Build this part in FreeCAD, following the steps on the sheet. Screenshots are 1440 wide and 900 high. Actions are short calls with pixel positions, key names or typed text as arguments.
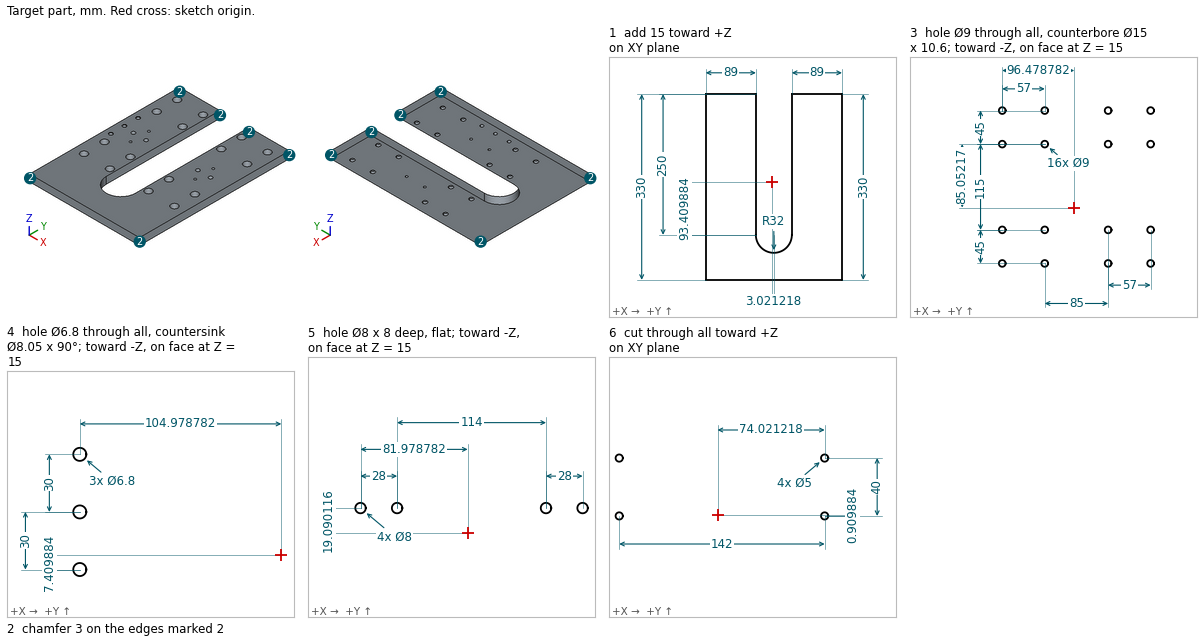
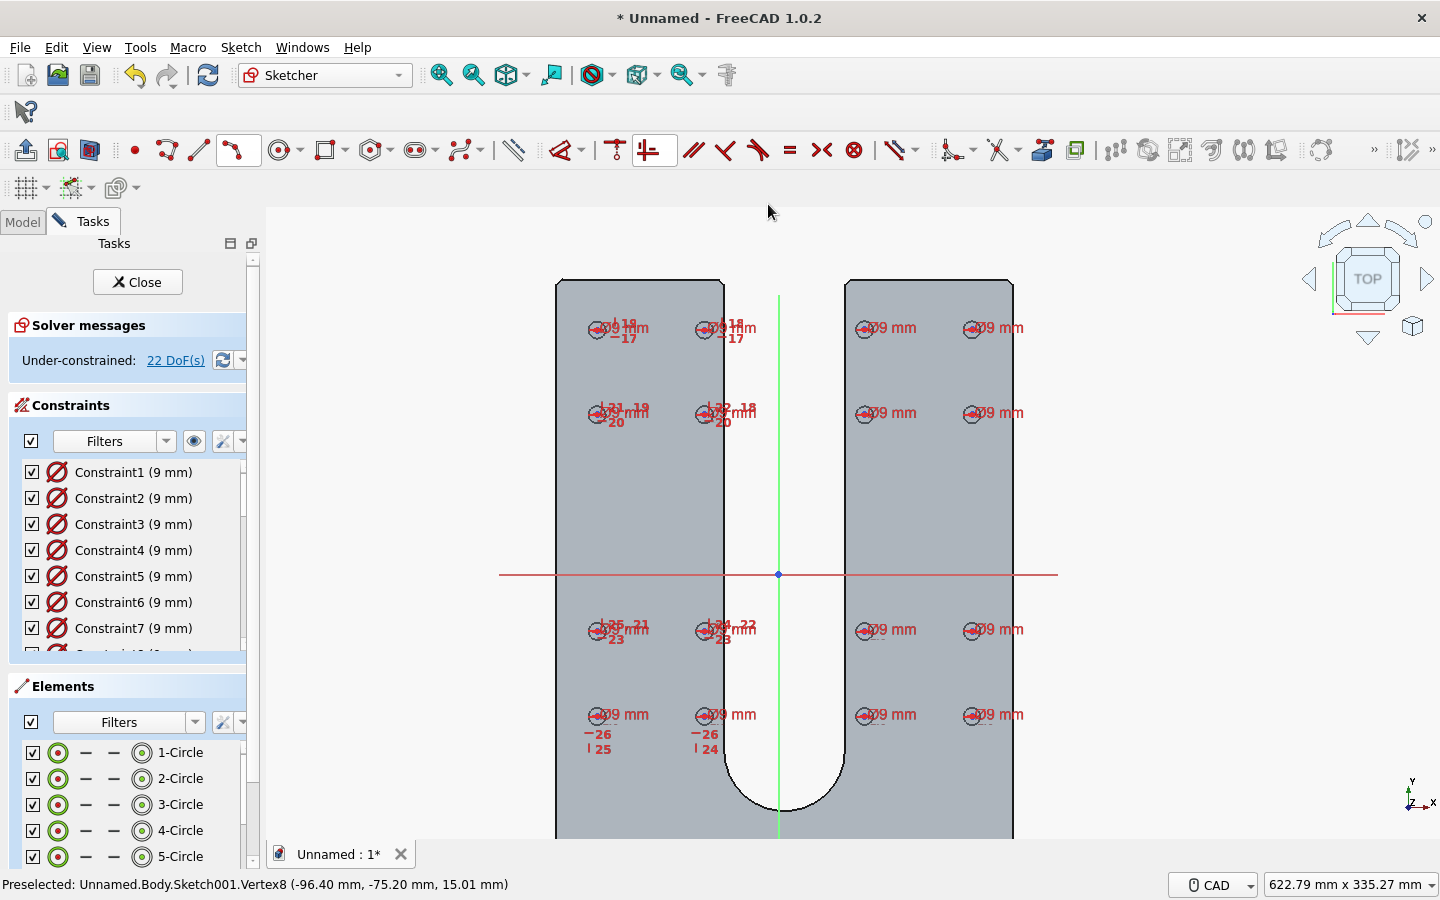
click(705, 717)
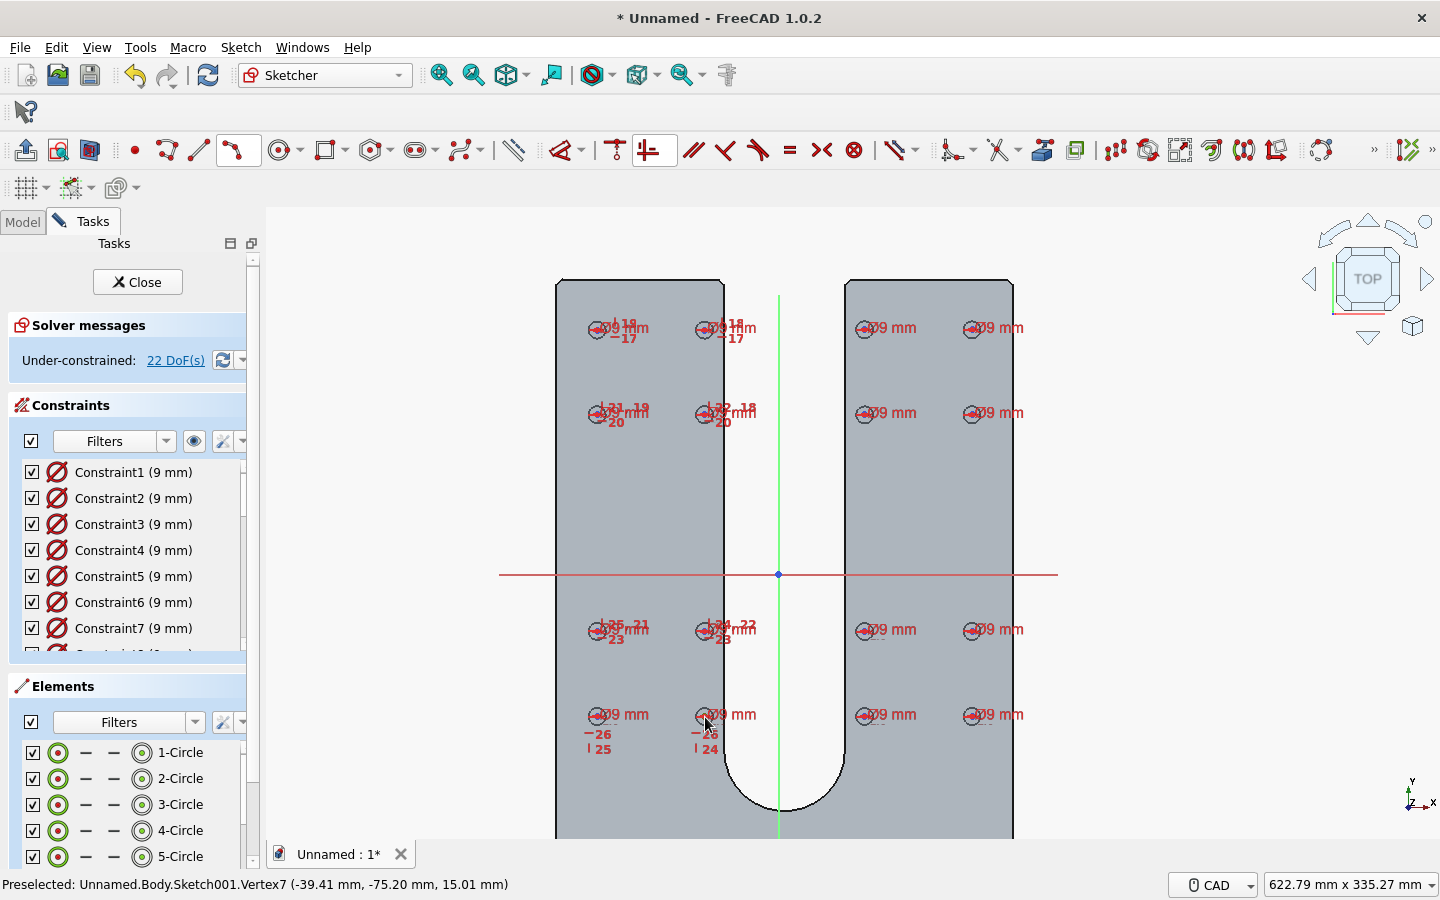
click(865, 717)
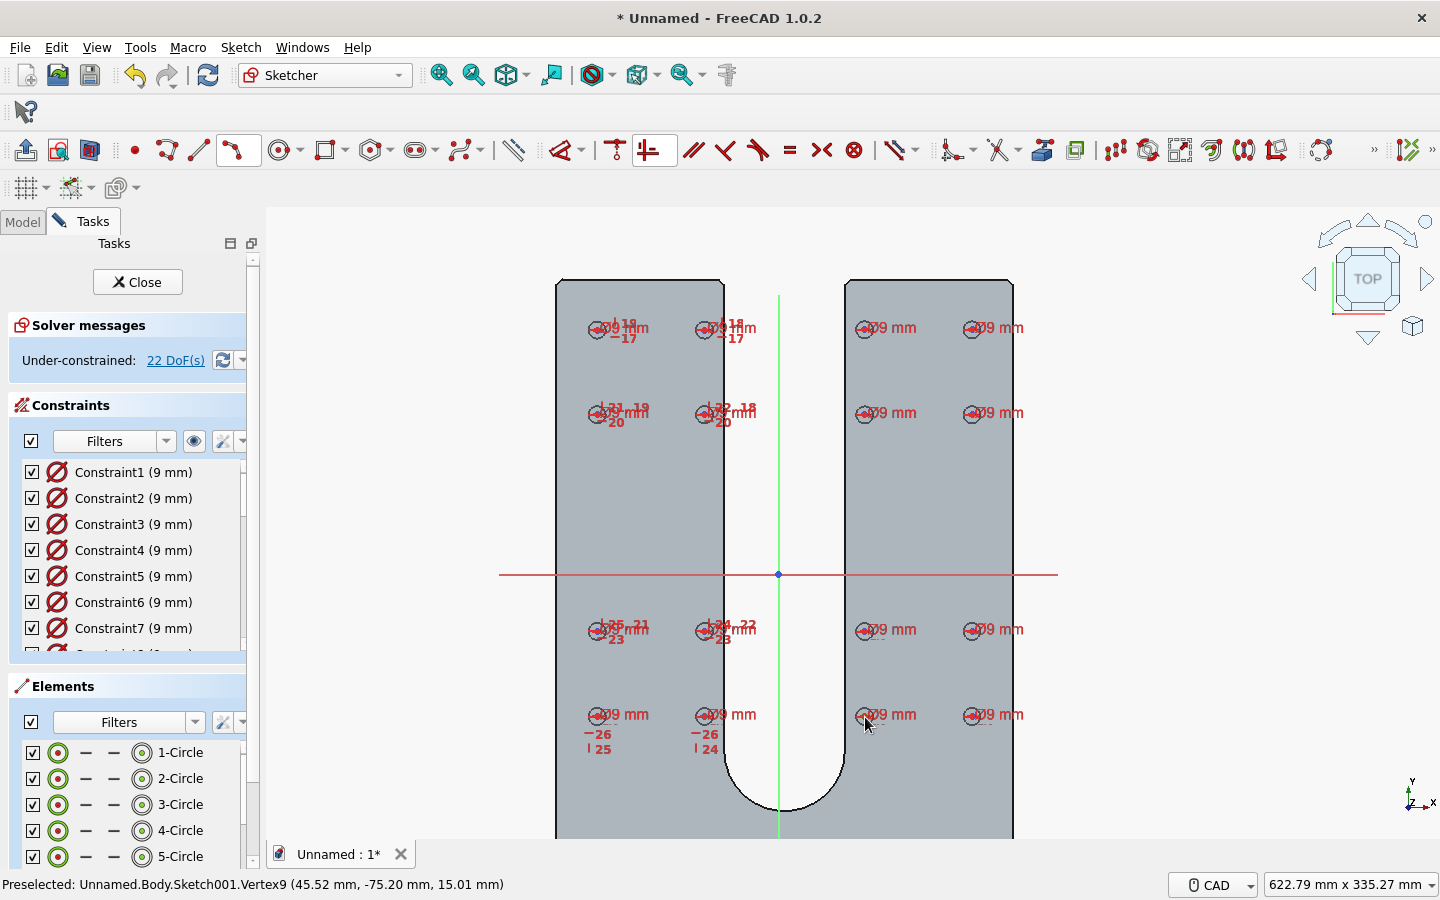
click(672, 150)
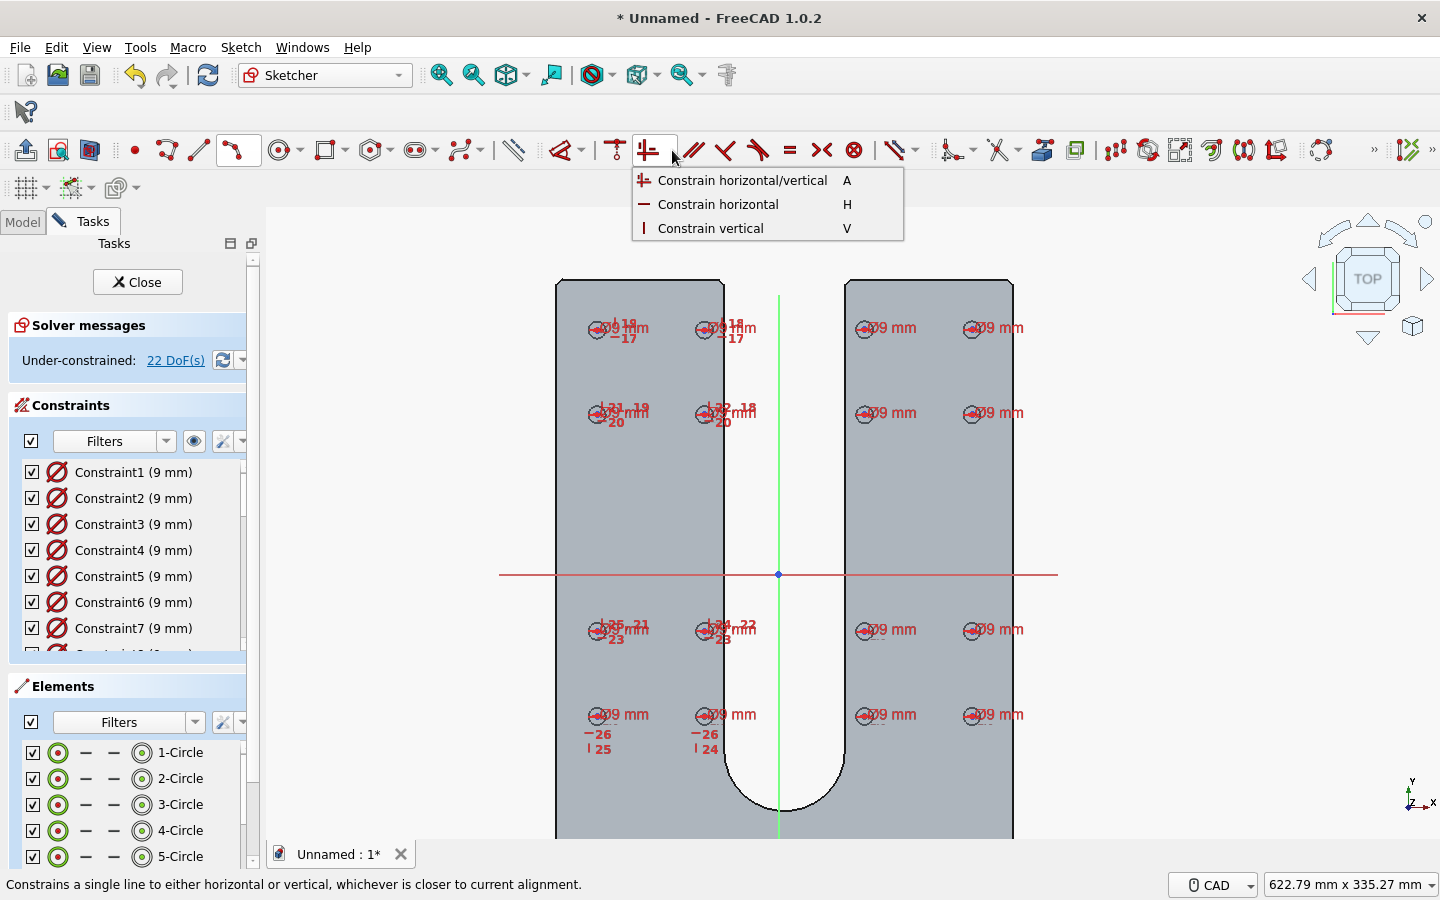
click(768, 204)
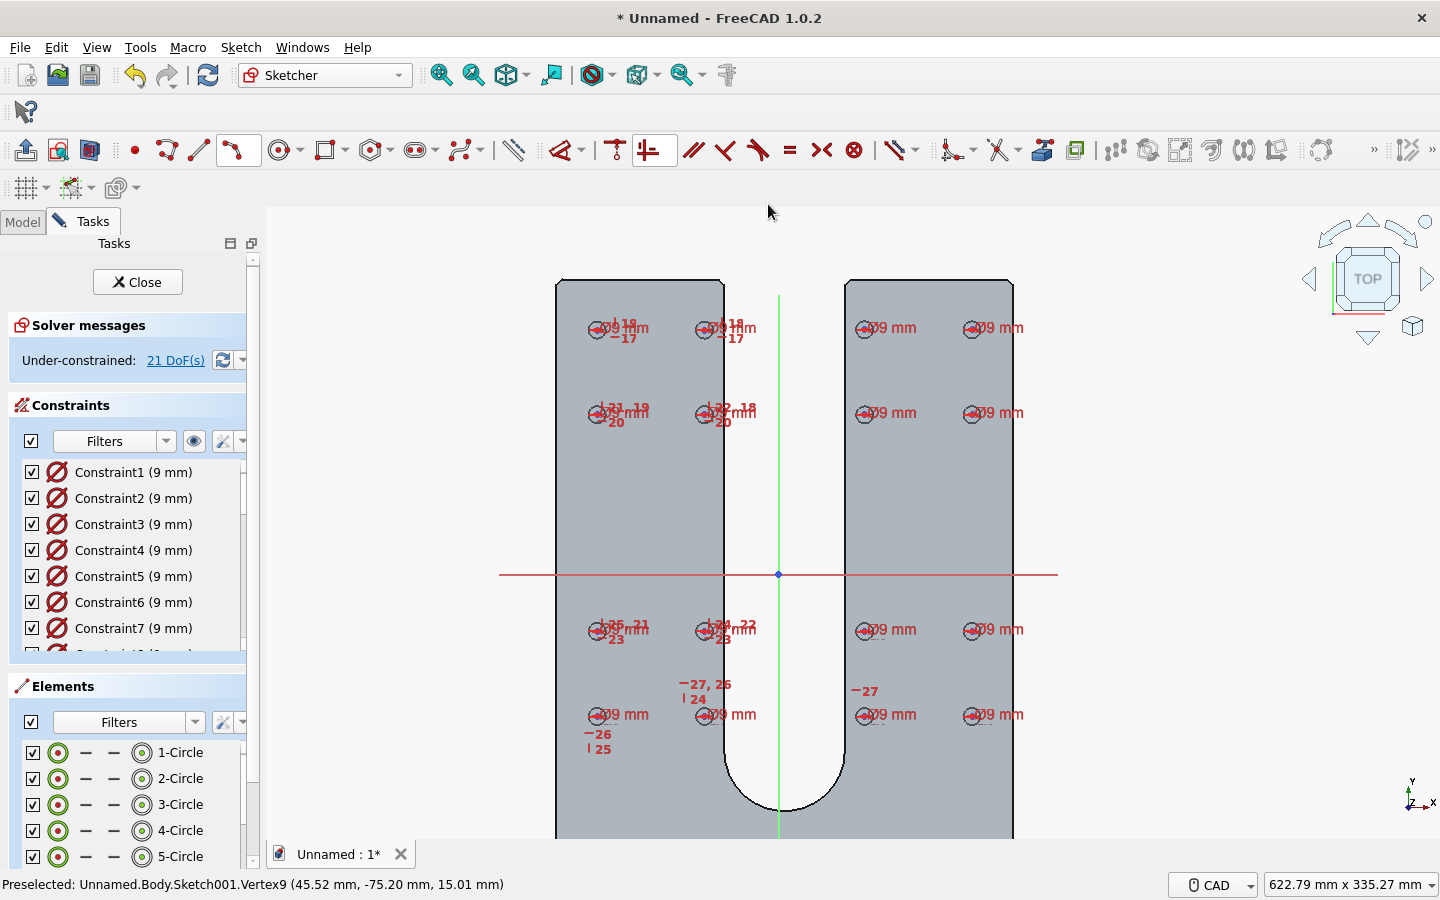
click(865, 717)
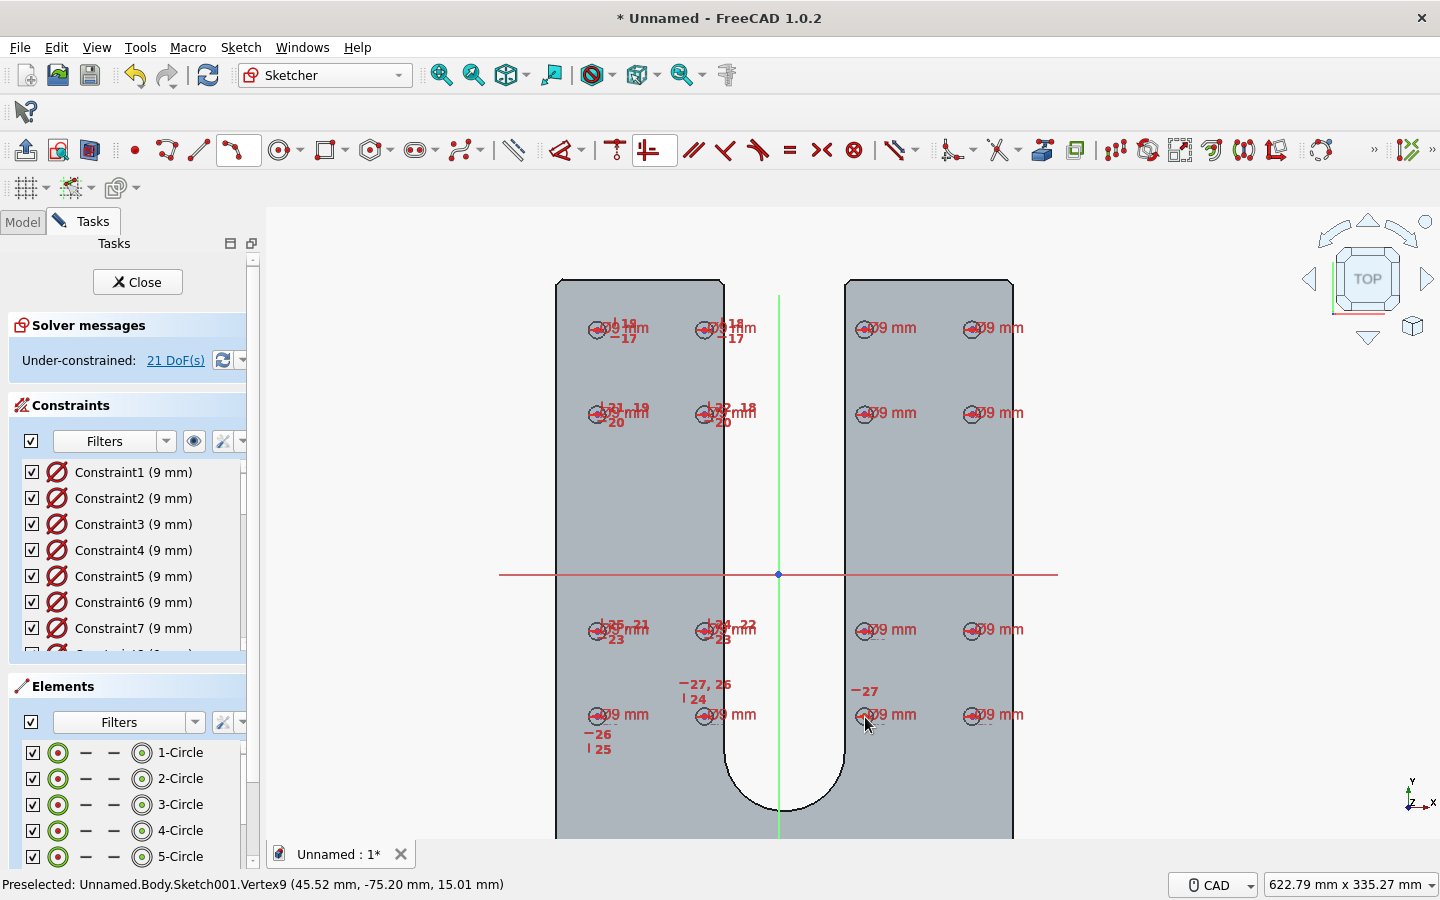
click(865, 632)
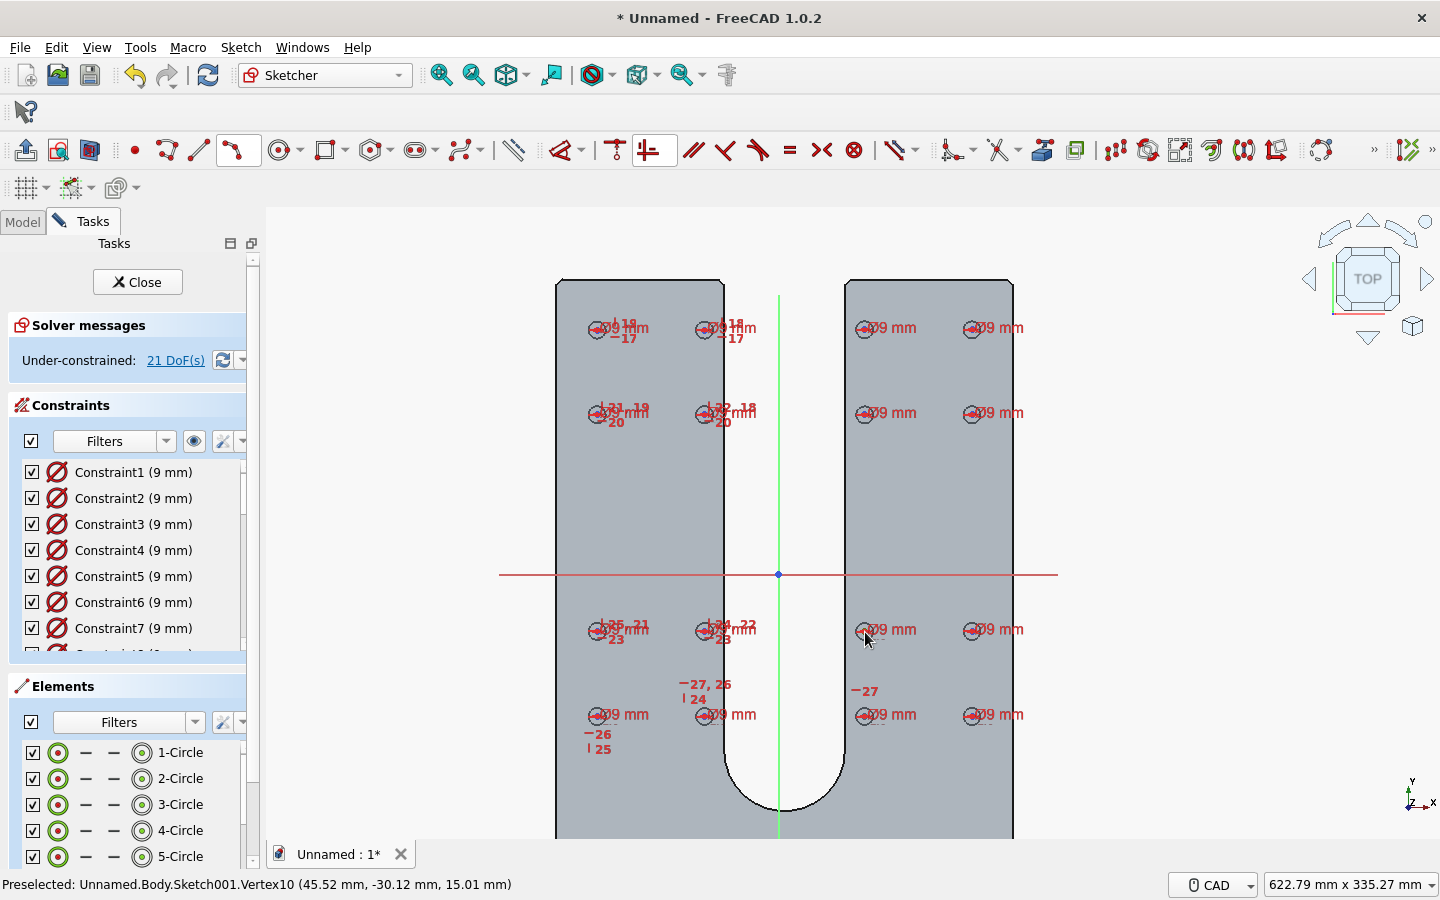
click(672, 150)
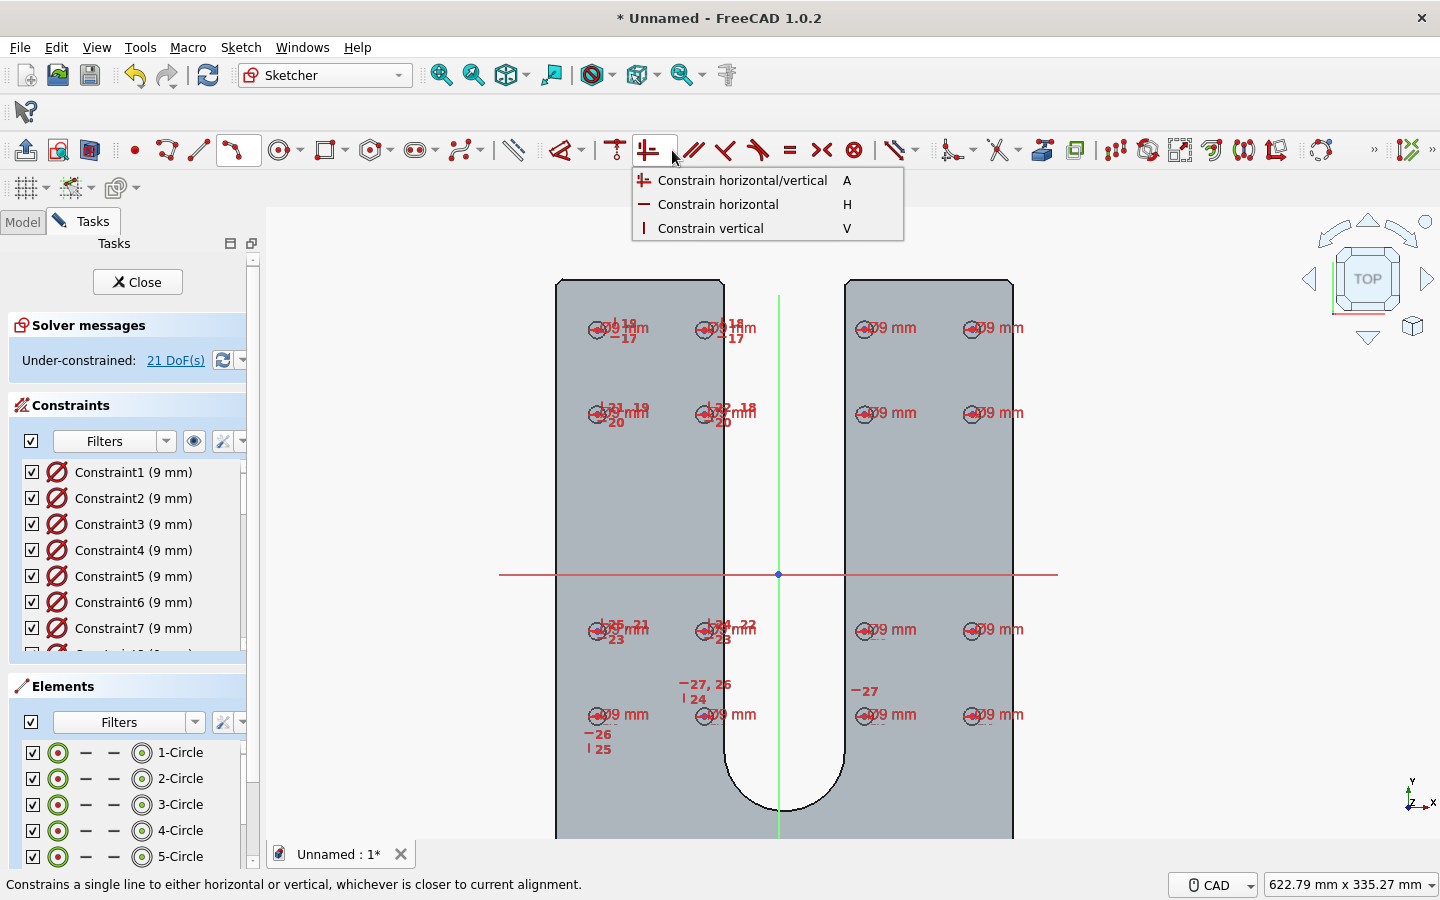
click(768, 228)